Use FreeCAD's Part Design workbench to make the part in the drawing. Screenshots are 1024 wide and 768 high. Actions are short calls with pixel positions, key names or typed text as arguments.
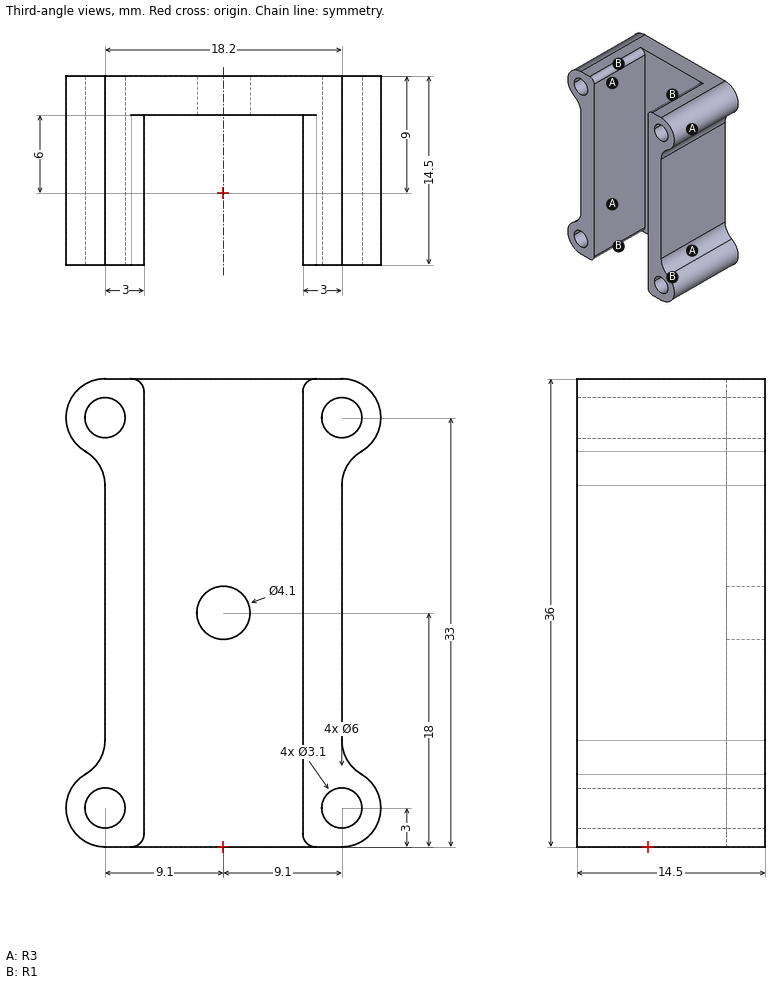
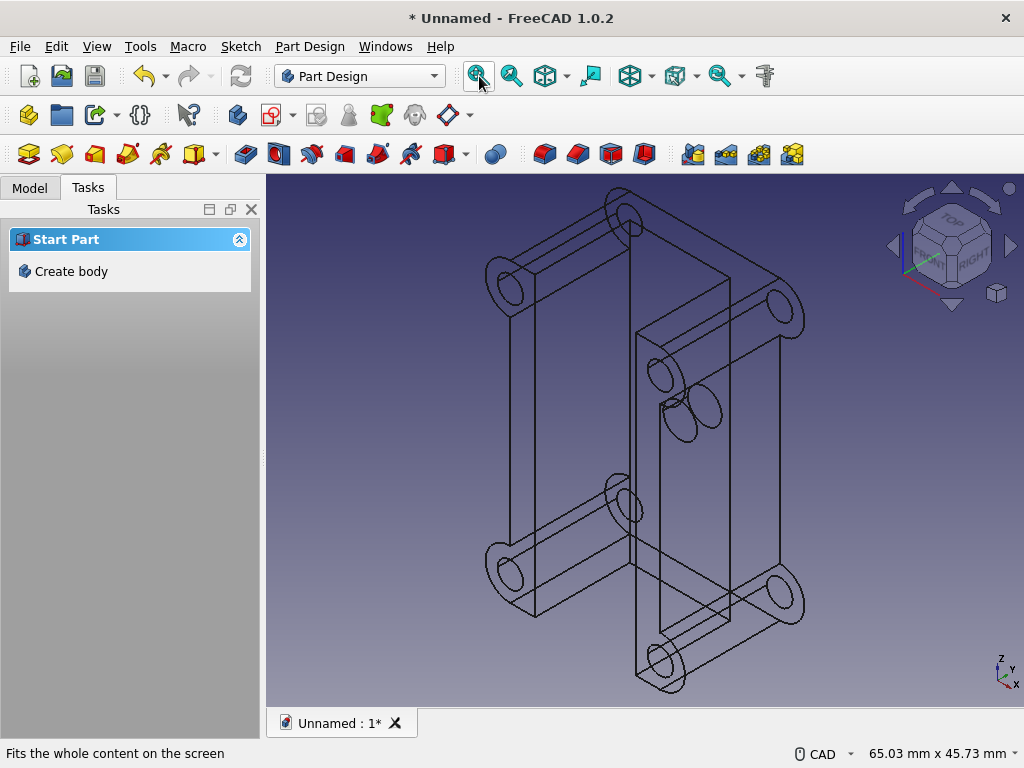
click(720, 597)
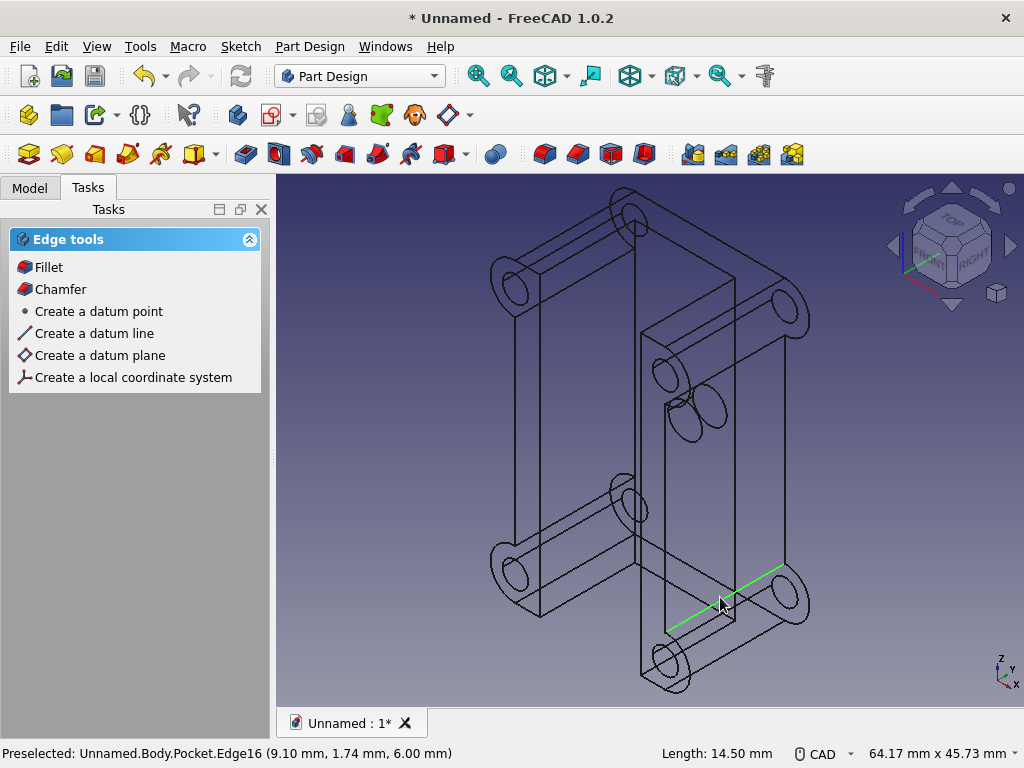
click(575, 510, ctrl)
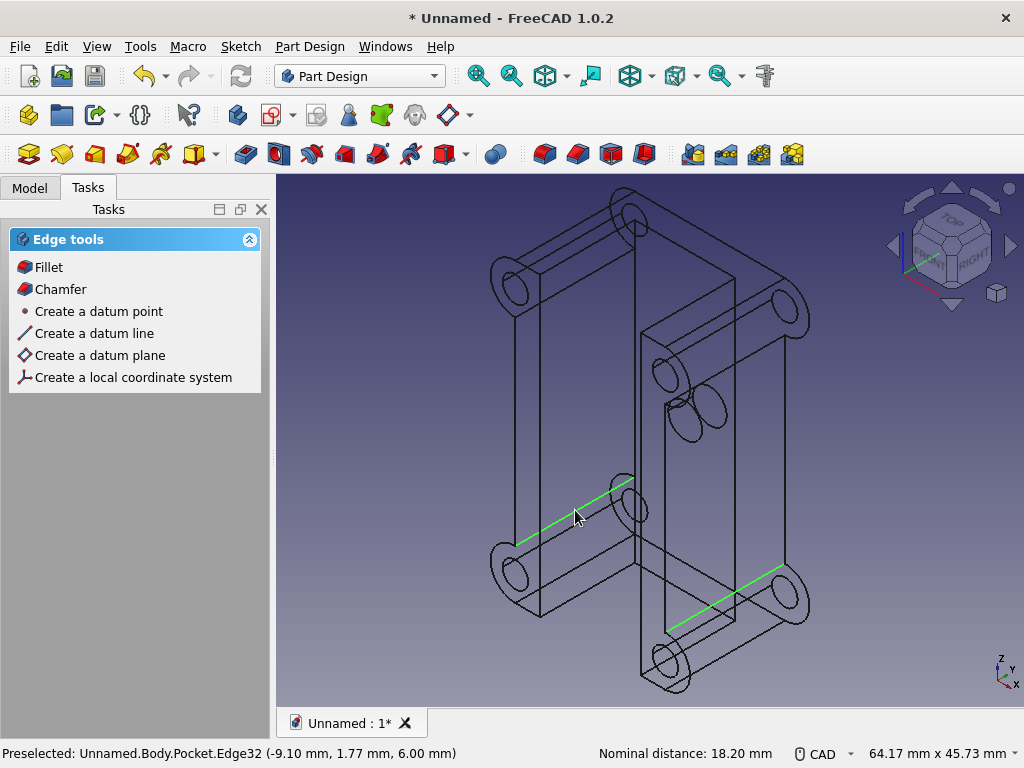
click(725, 369, ctrl)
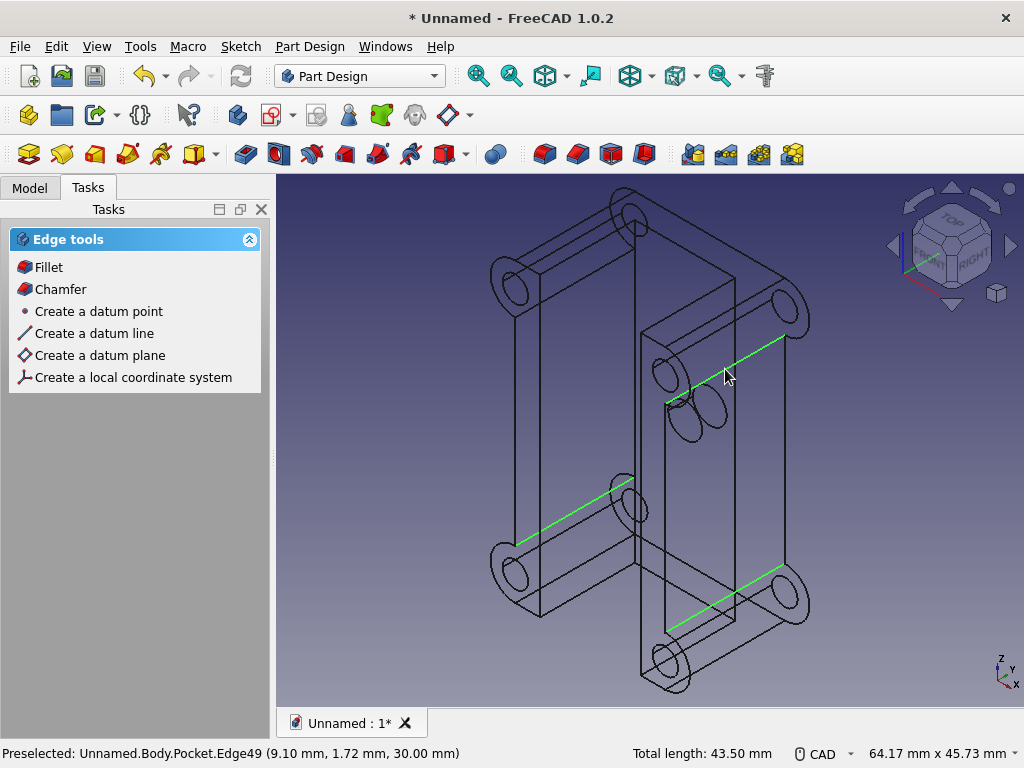
click(575, 282, ctrl)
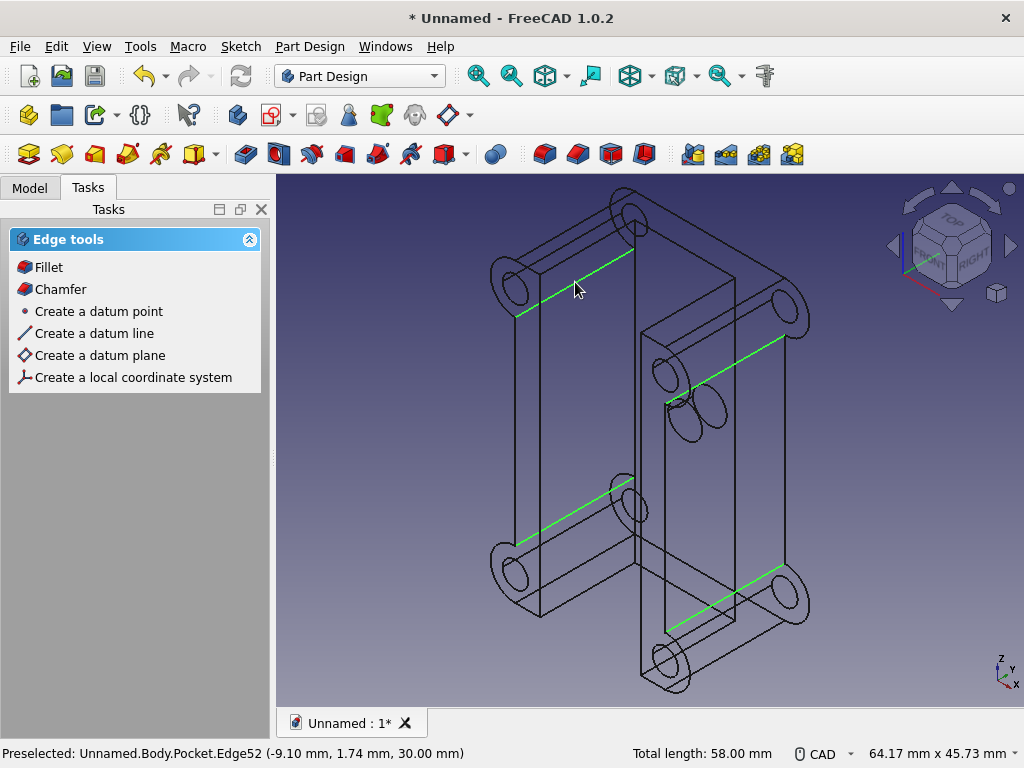
key(v)
key(1)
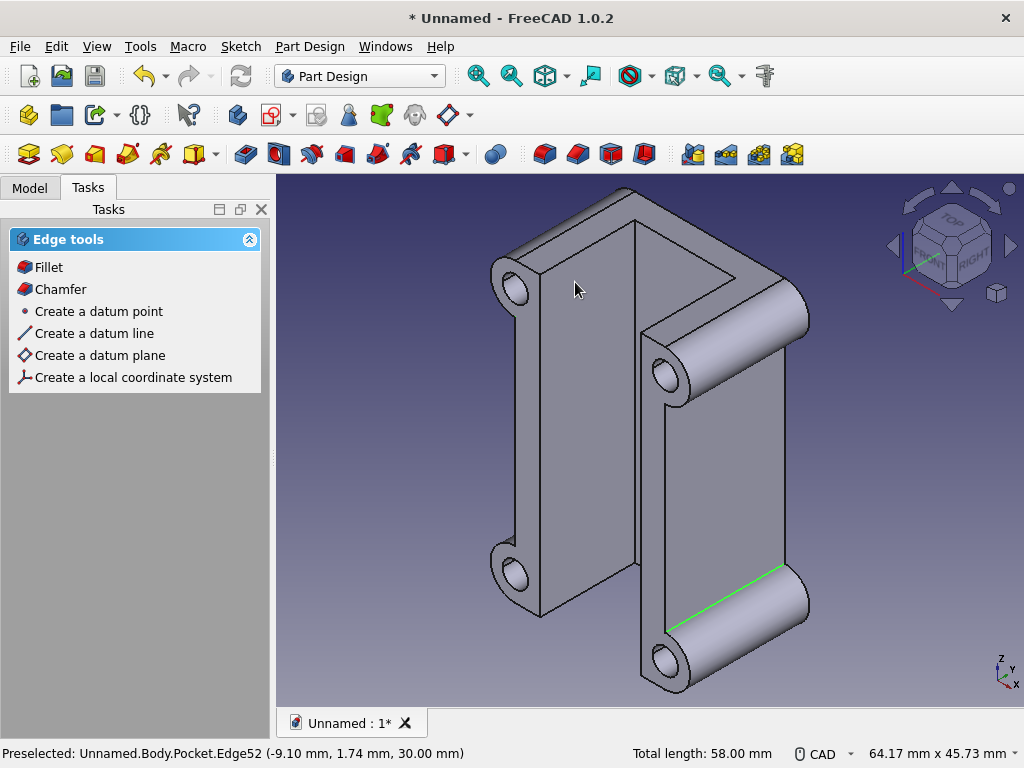
click(545, 154)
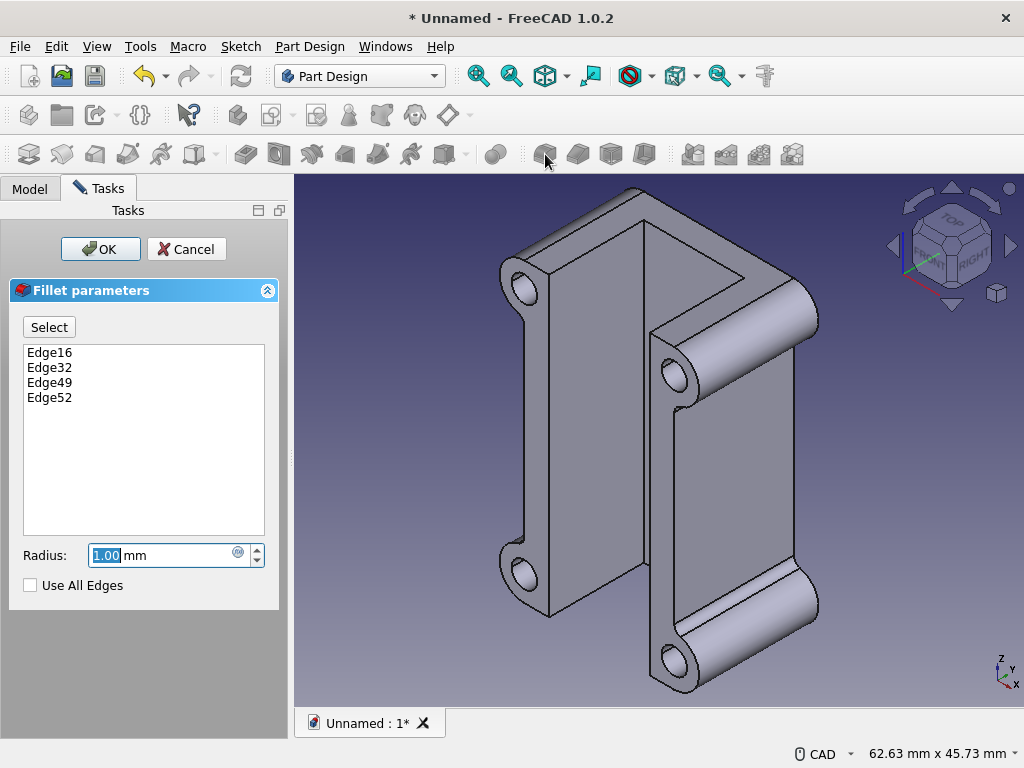
text(3)
key(Tab)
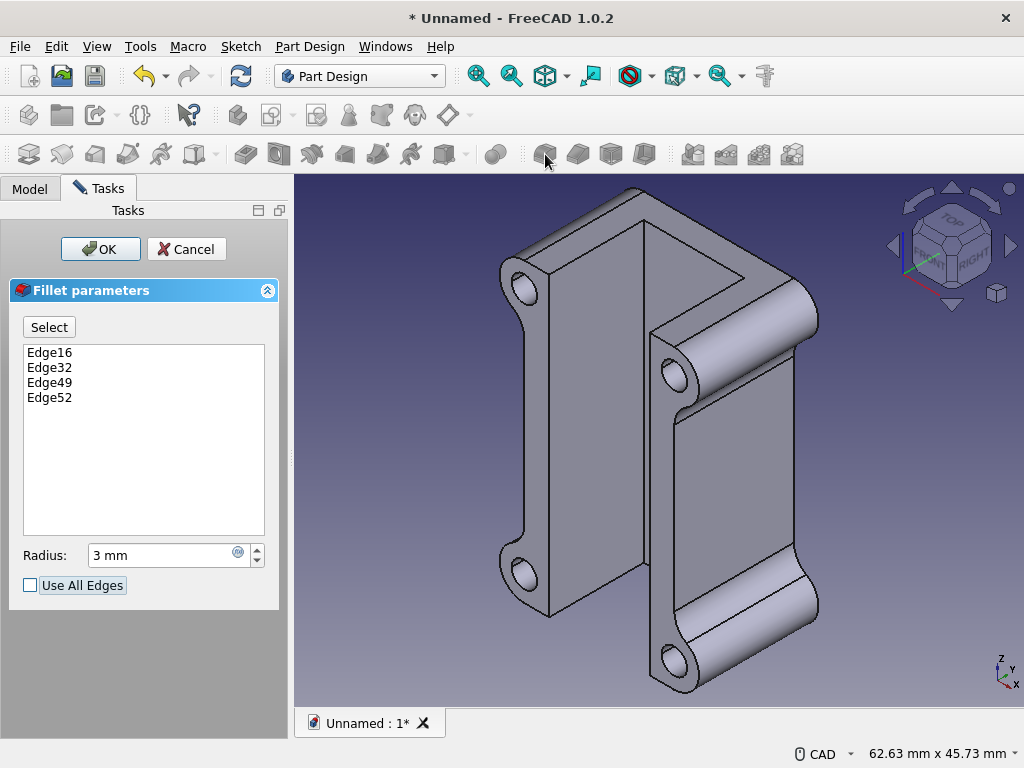
click(101, 249)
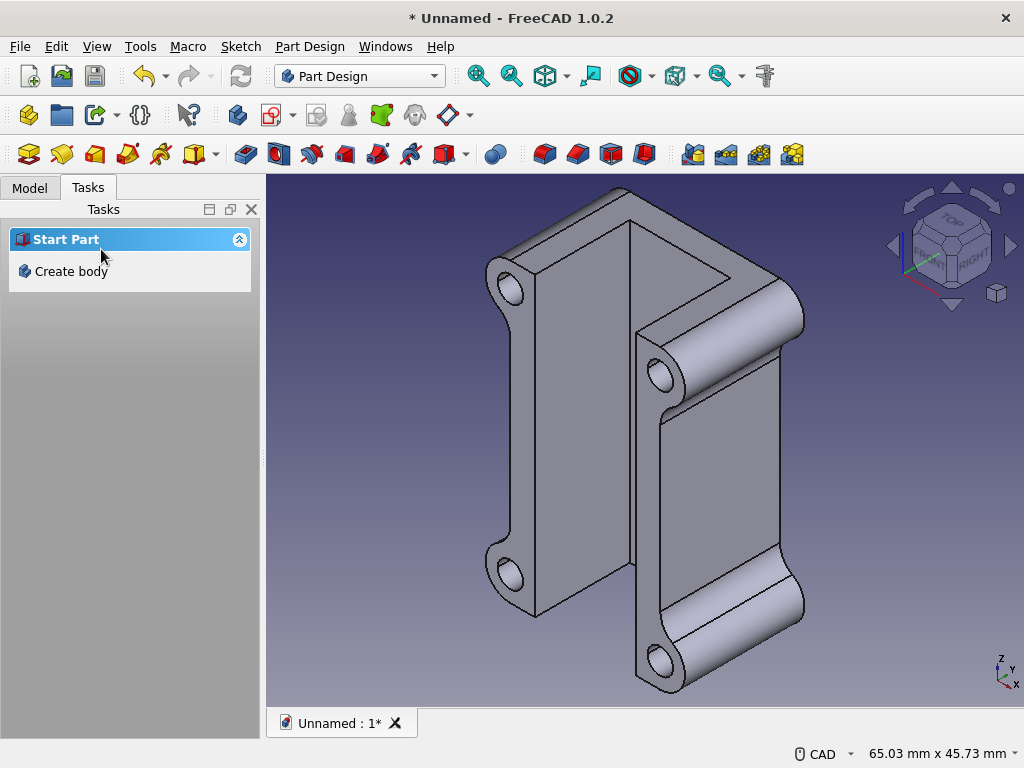
click(582, 246)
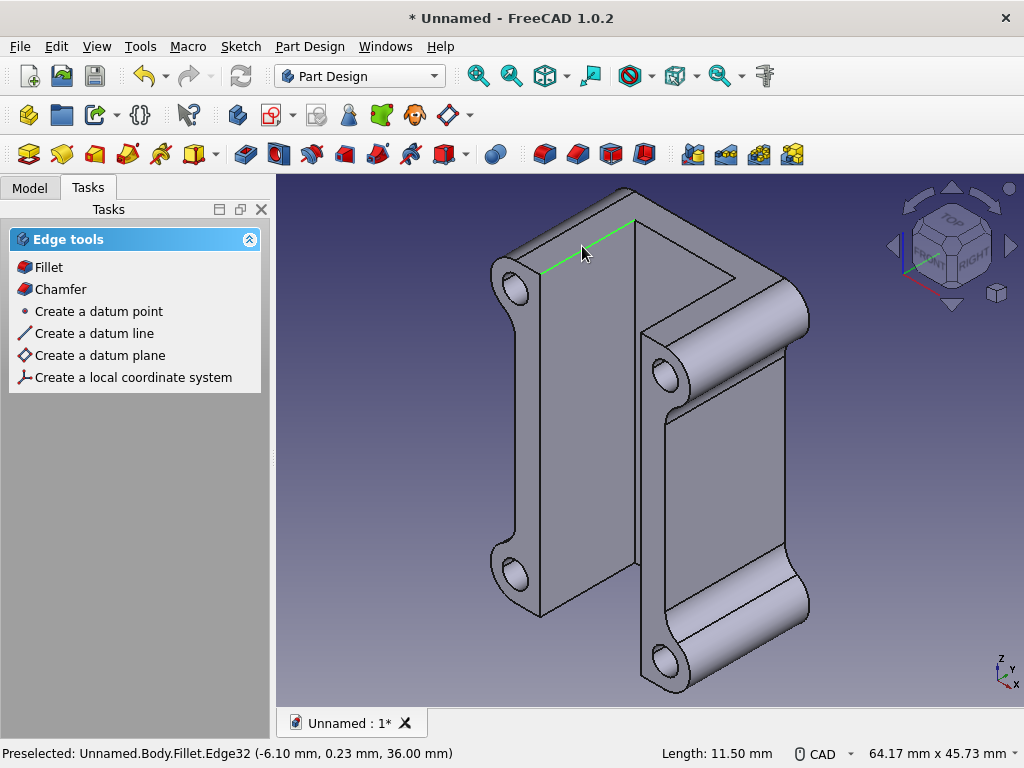
key(2)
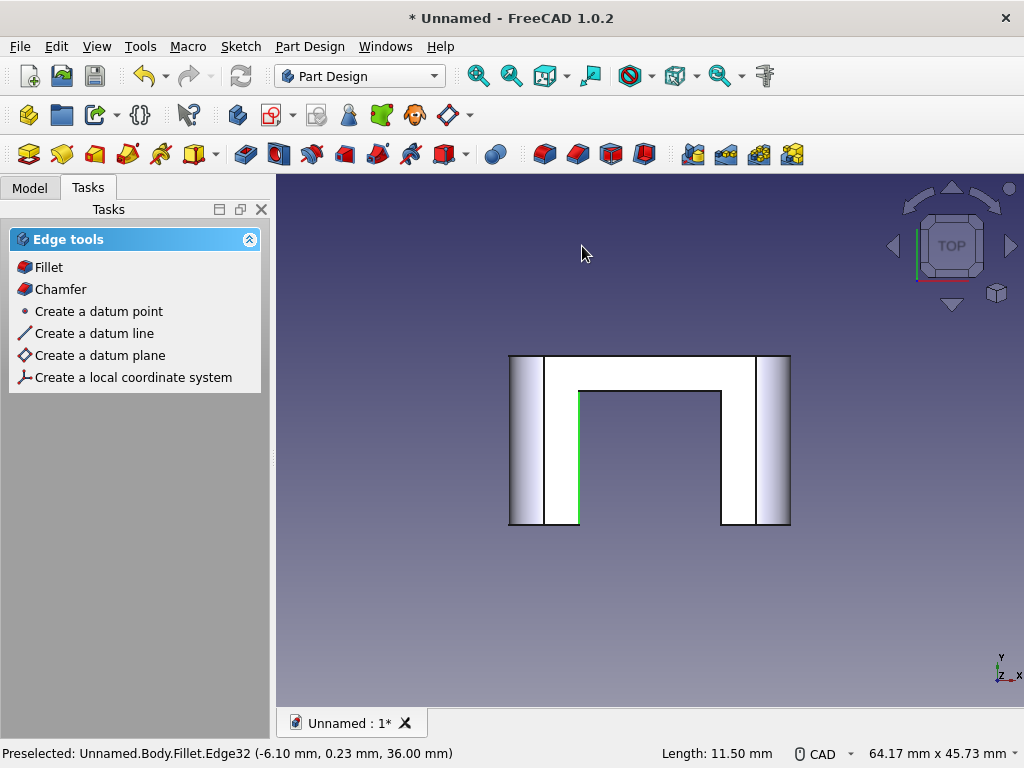
click(479, 76)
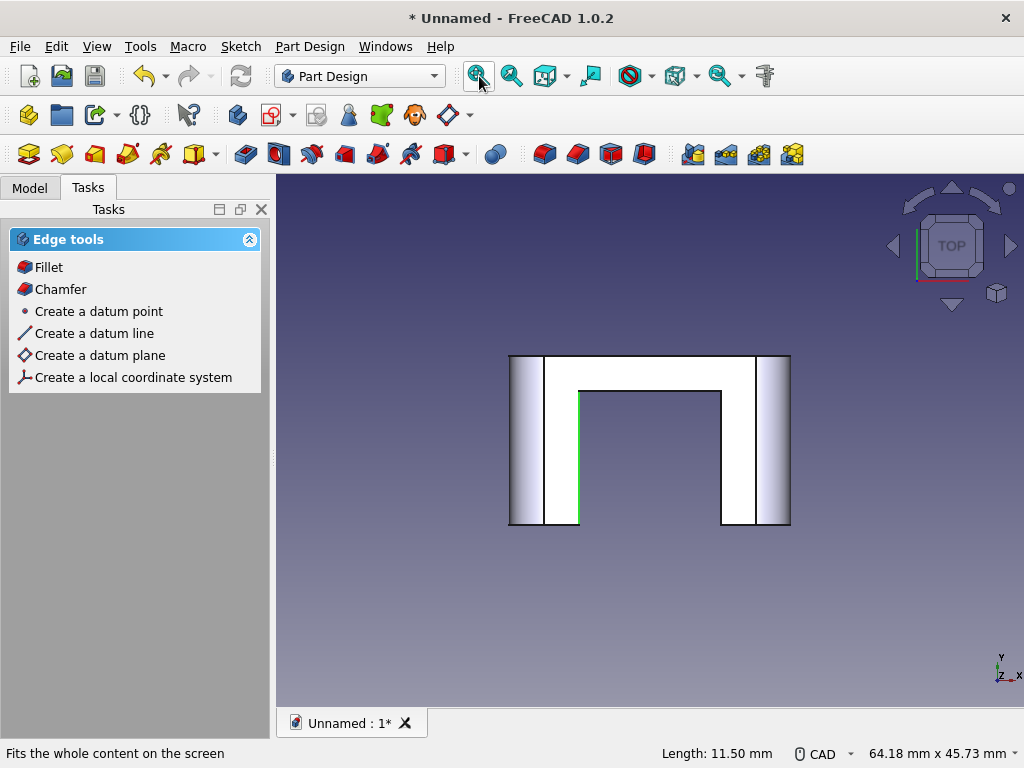
click(721, 457, ctrl)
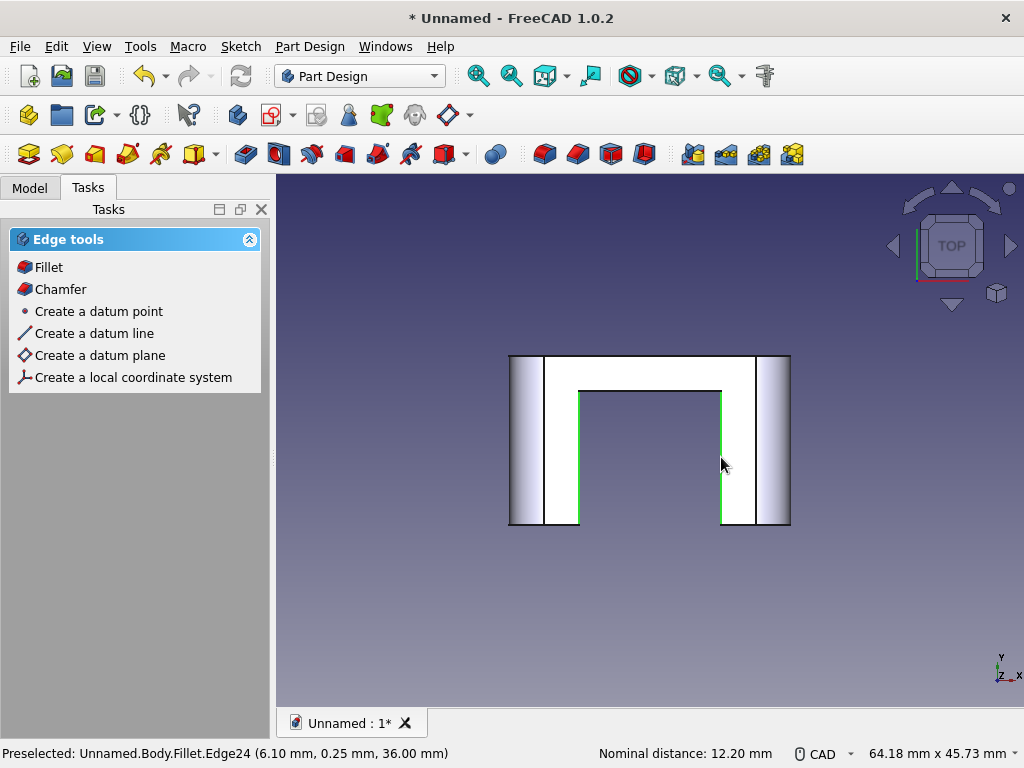
key(0)